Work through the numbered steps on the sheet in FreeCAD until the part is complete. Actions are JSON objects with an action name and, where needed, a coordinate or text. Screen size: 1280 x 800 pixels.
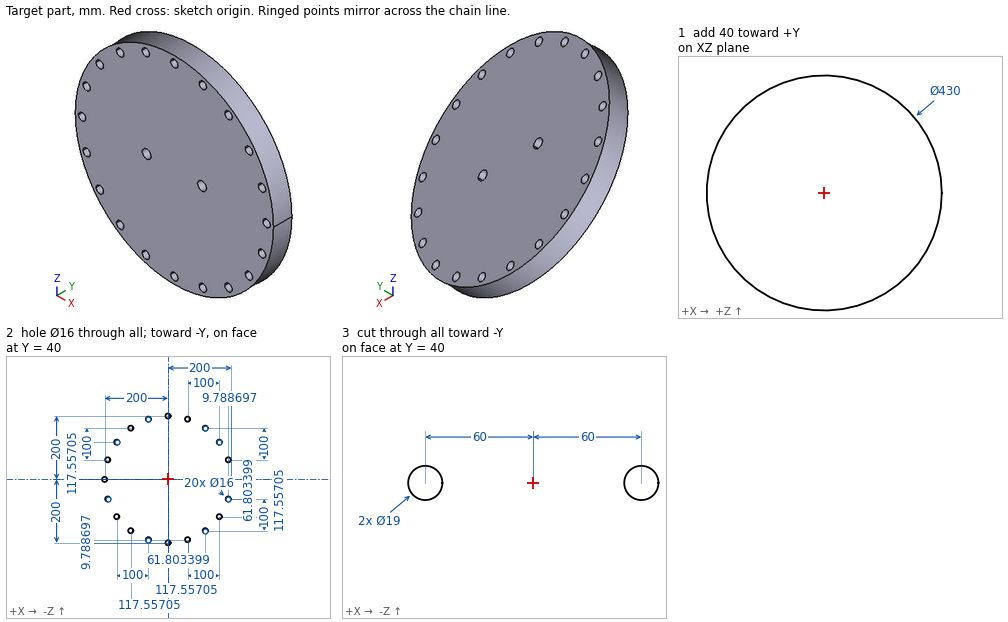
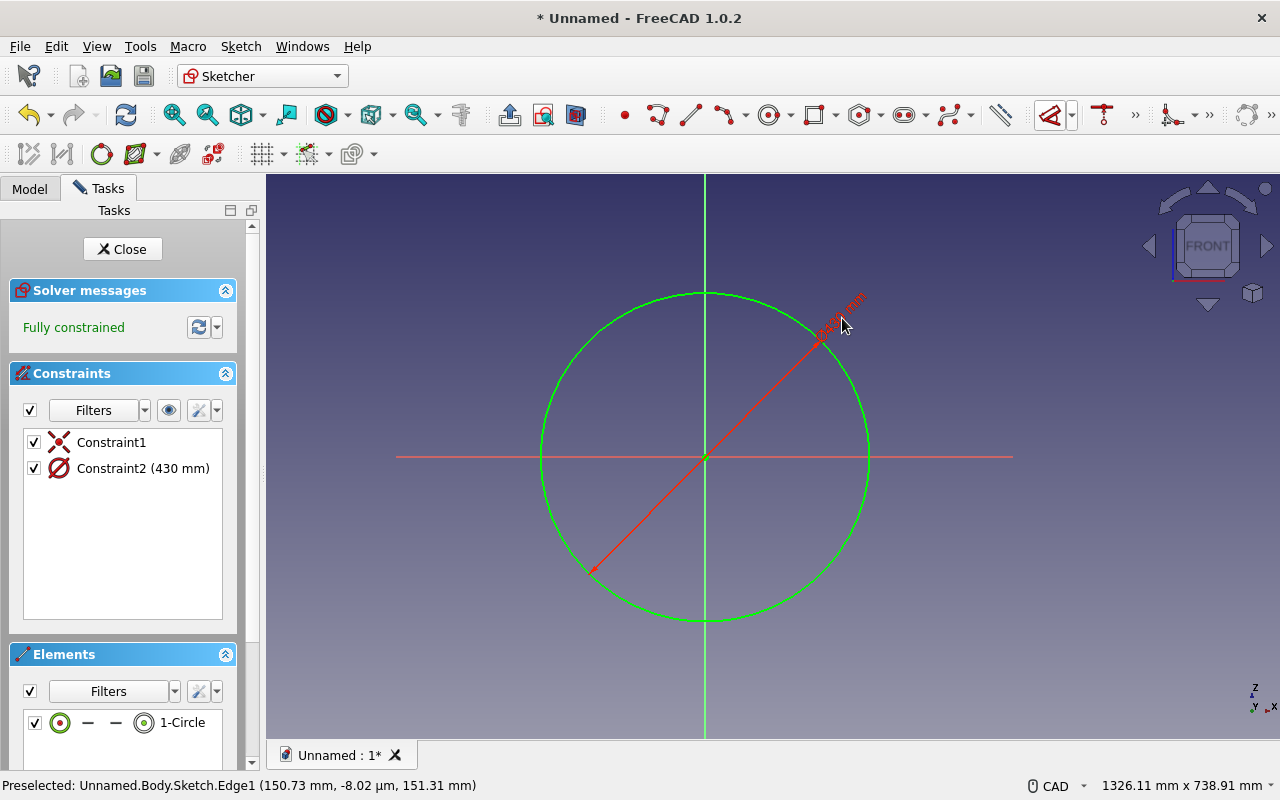
{"action": "left_click", "coordinate": [123, 249]}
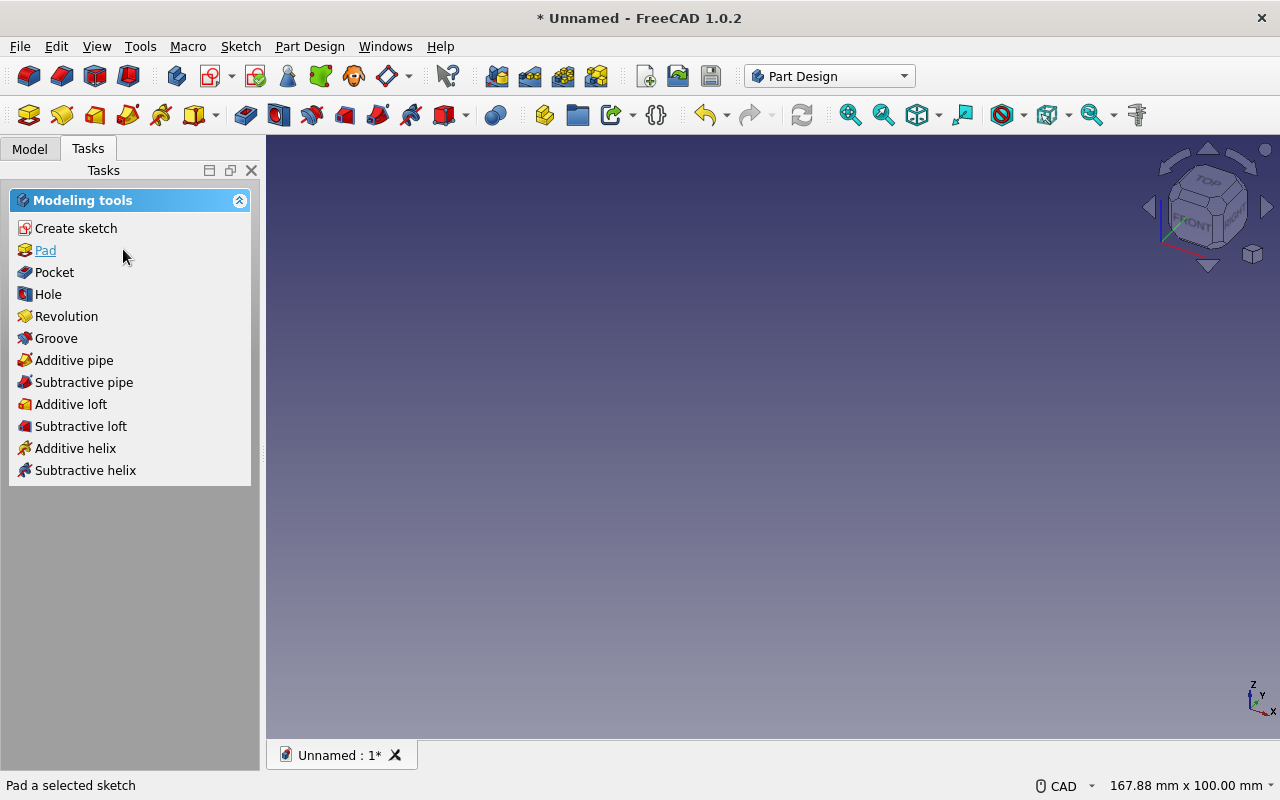
{"action": "left_click", "coordinate": [29, 116]}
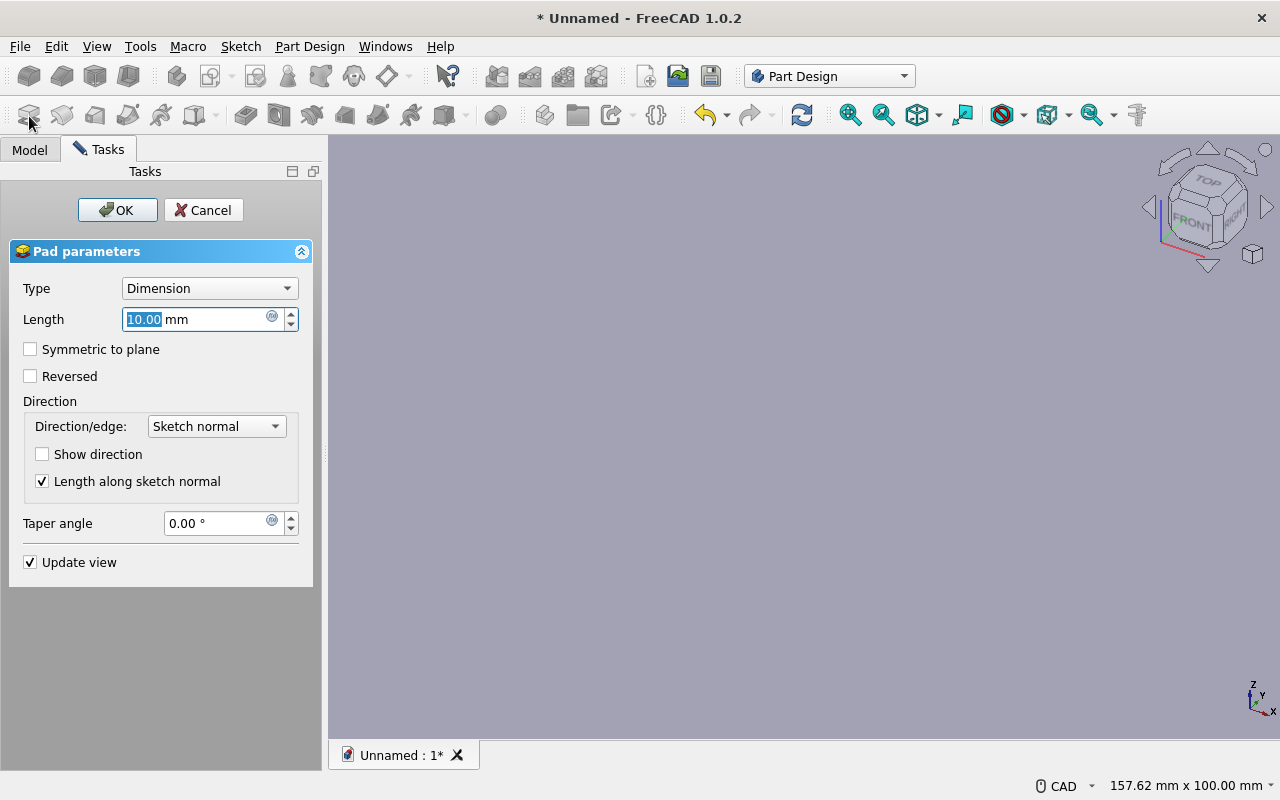
{"action": "type", "text": "40"}
{"action": "key", "text": "Tab"}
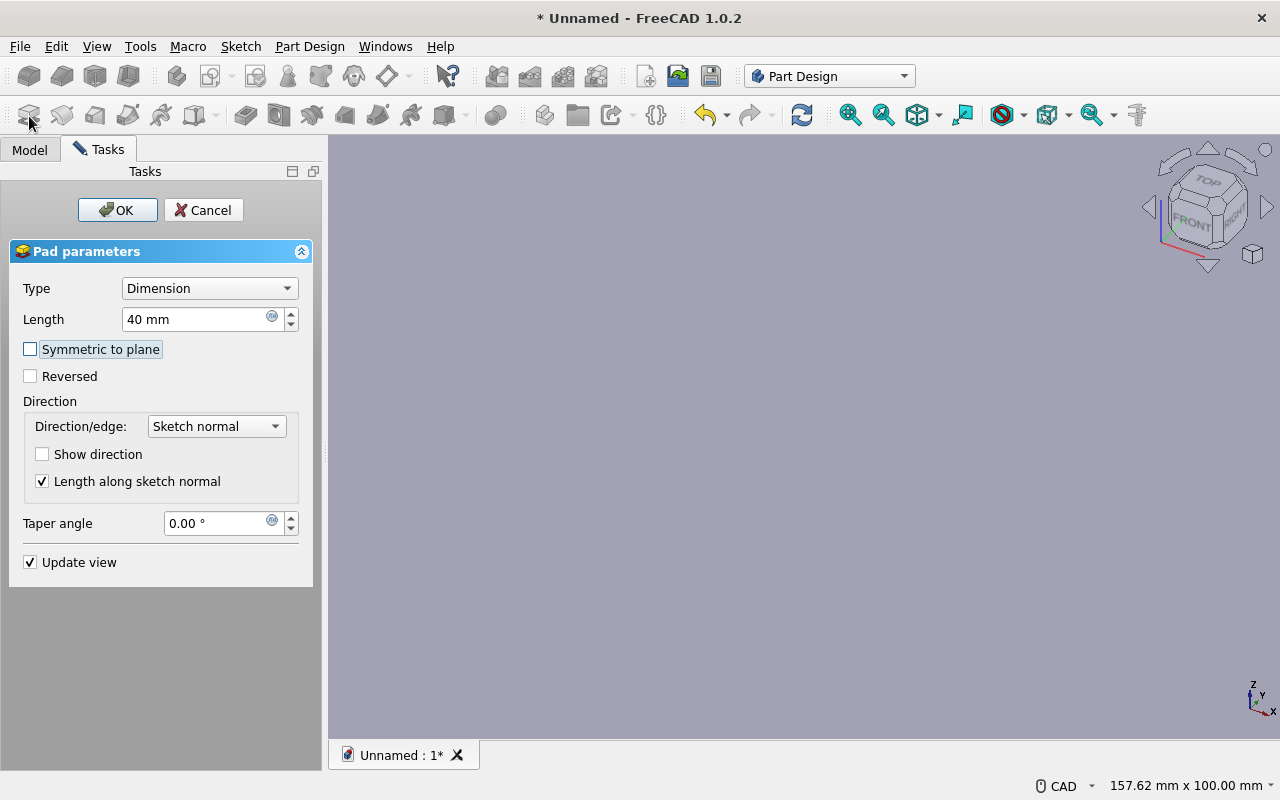
{"action": "left_click", "coordinate": [31, 376]}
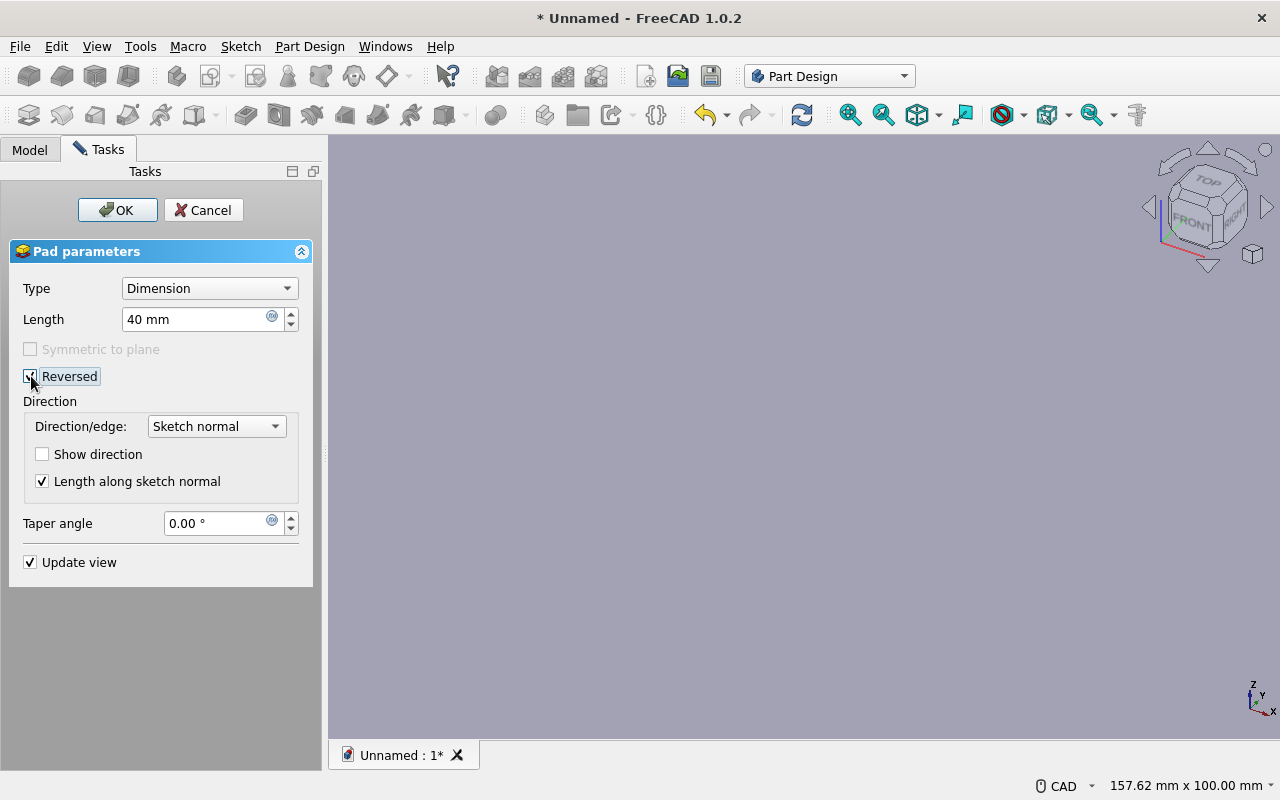
{"action": "left_click", "coordinate": [118, 210]}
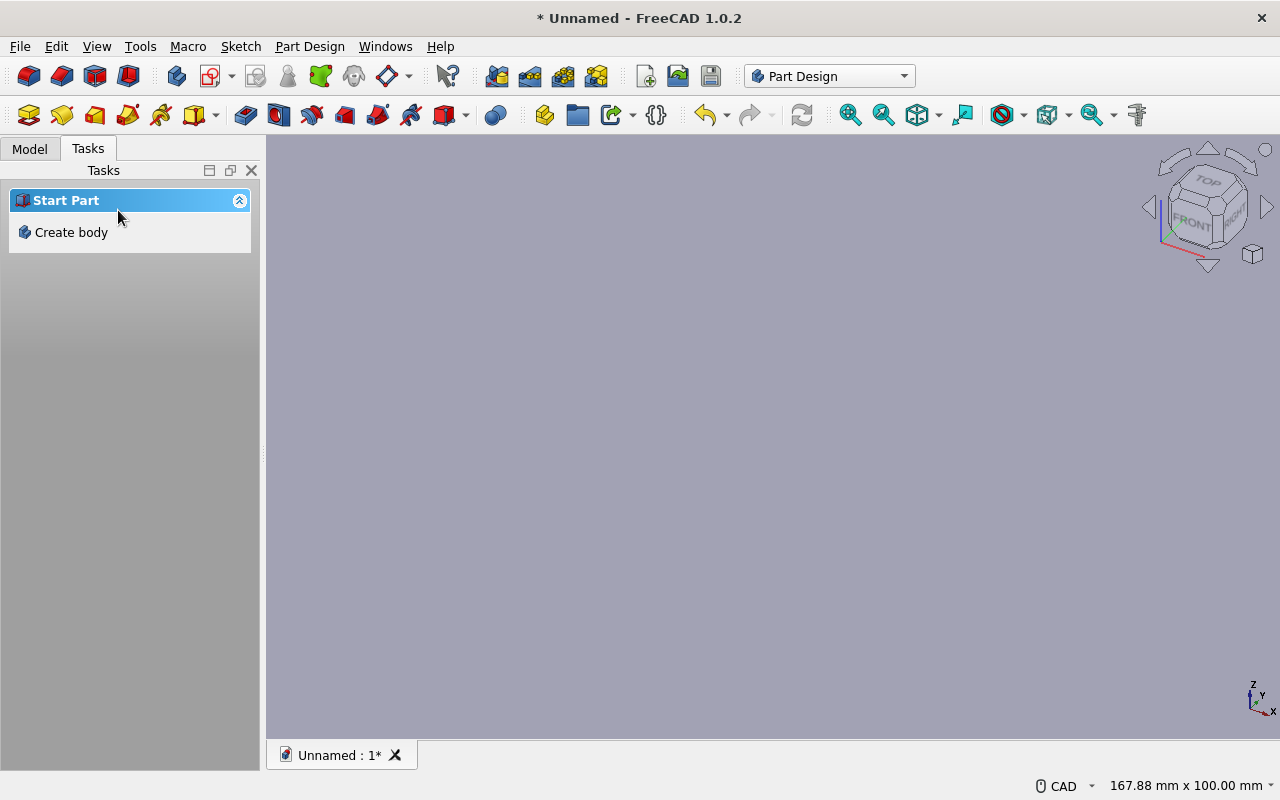
{"action": "left_click", "coordinate": [851, 116]}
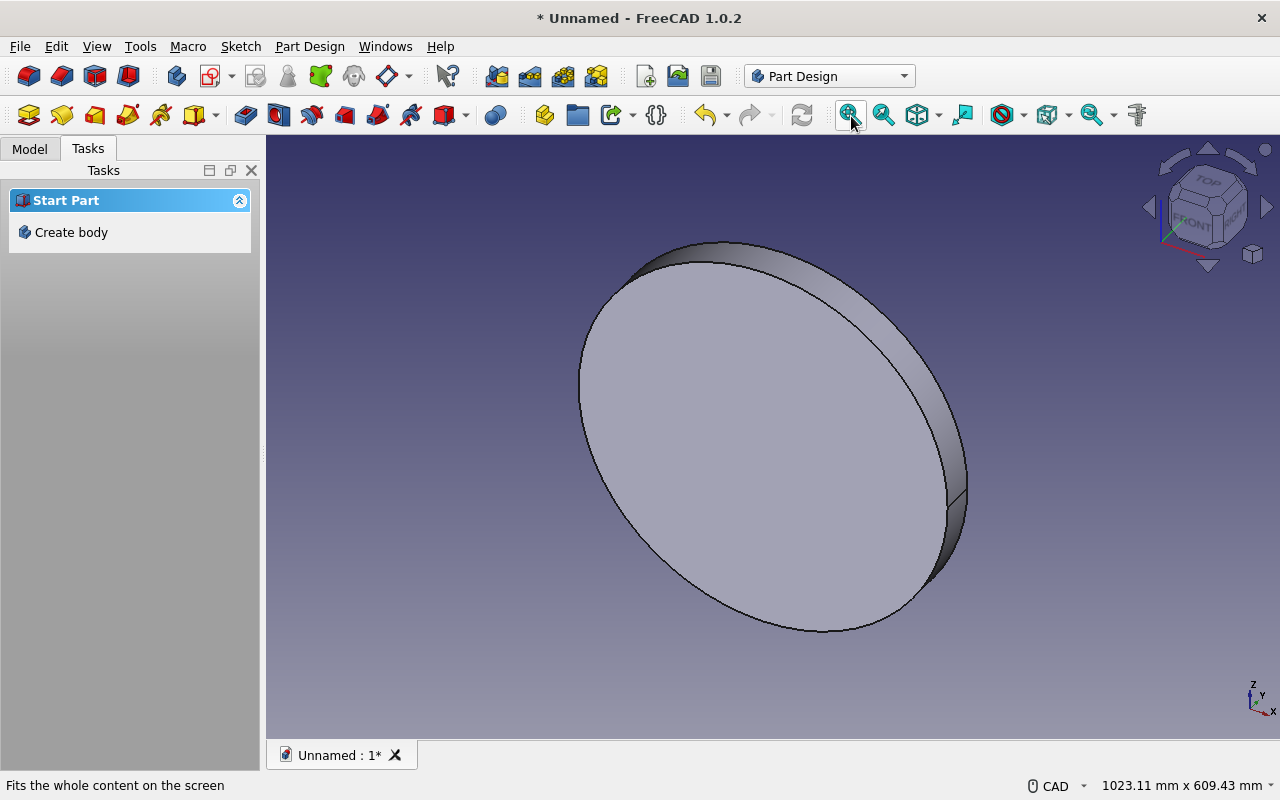
{"action": "key", "text": "4"}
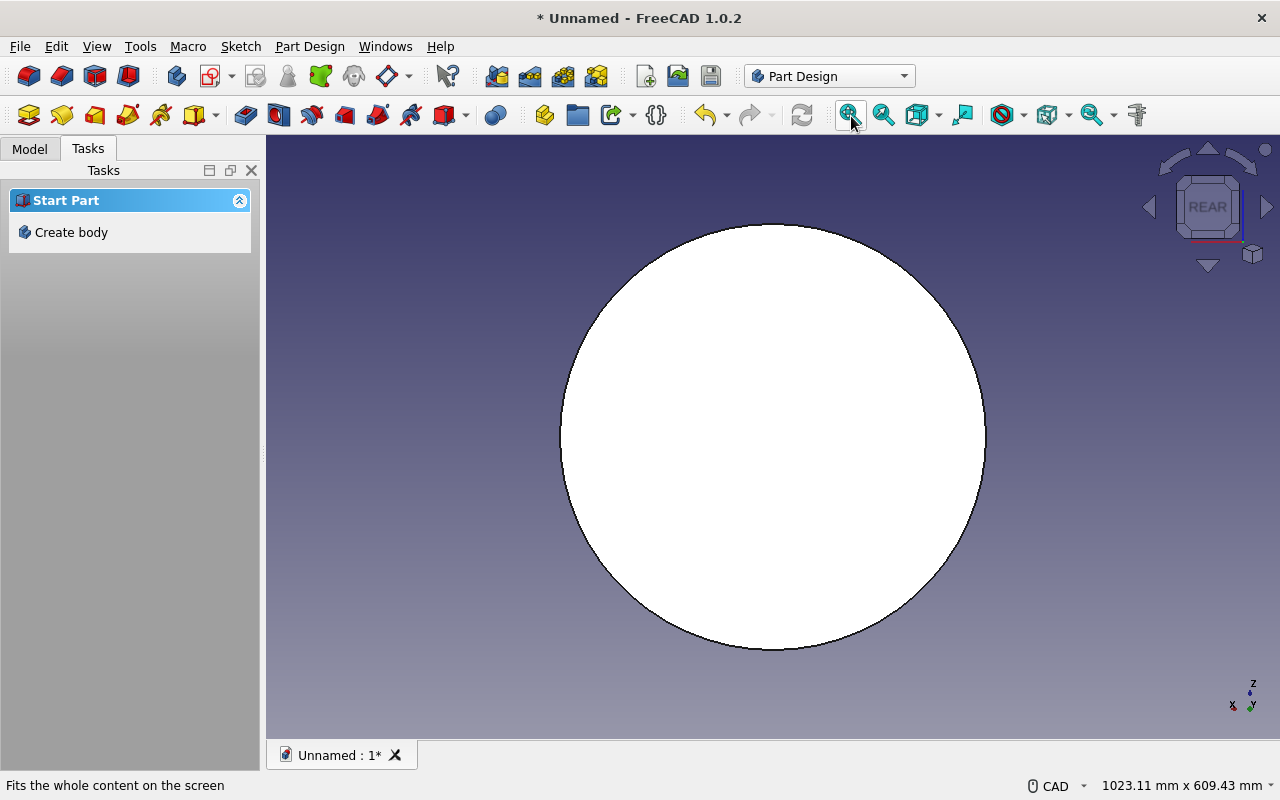
{"action": "left_click", "coordinate": [773, 436]}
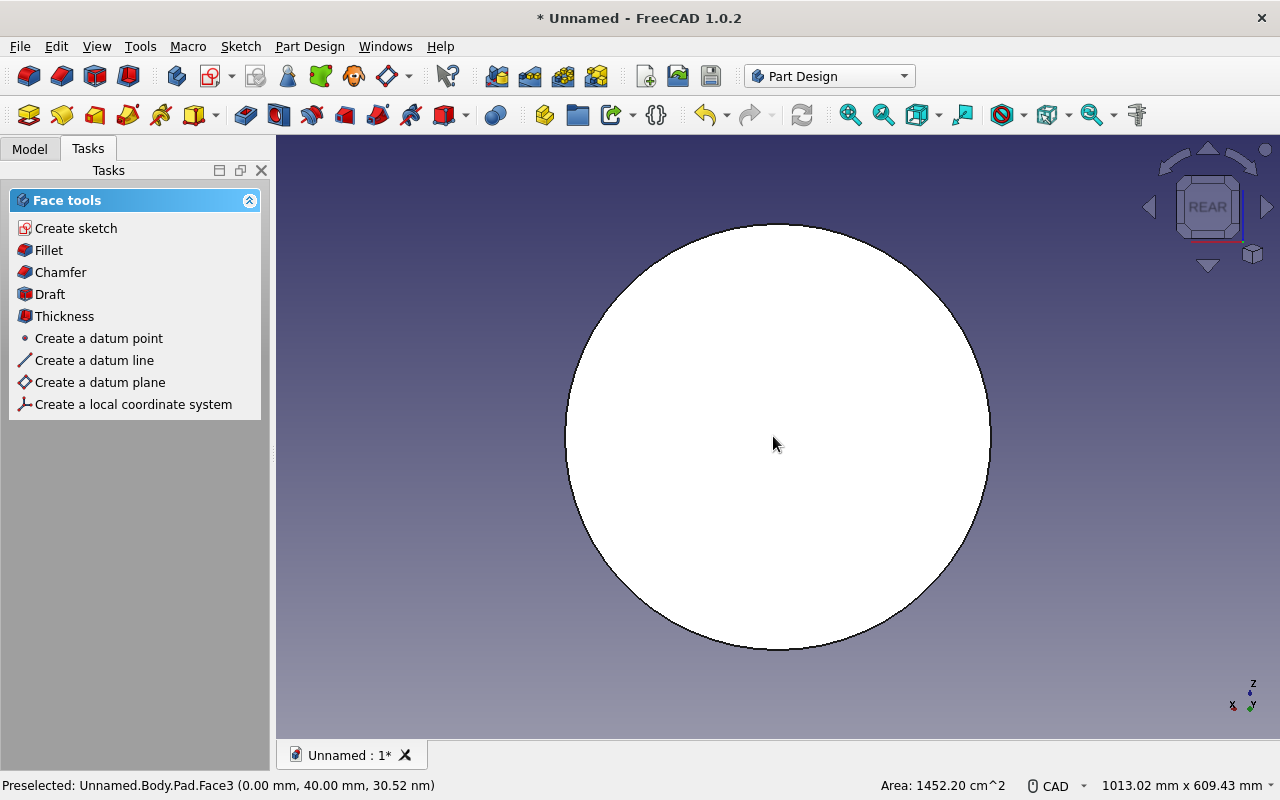
{"action": "left_click", "coordinate": [210, 76]}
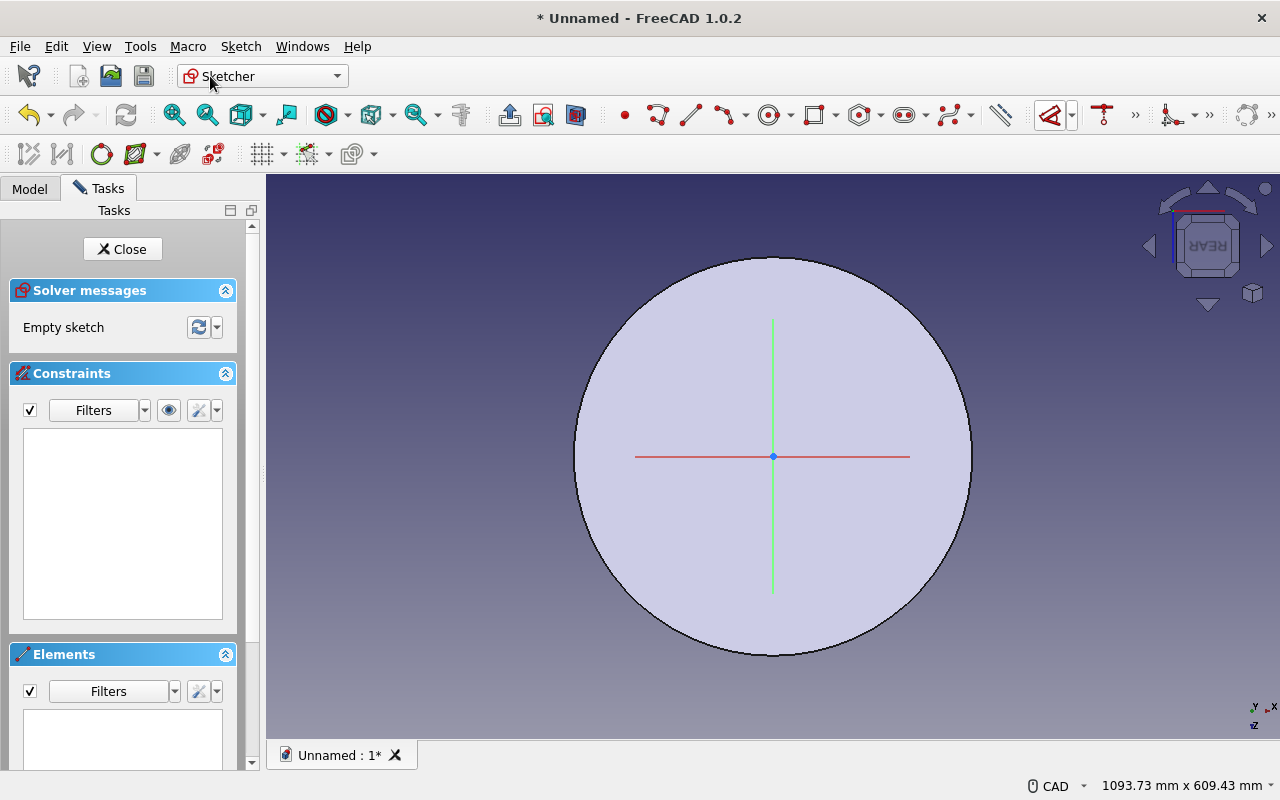
{"action": "left_click", "coordinate": [768, 116]}